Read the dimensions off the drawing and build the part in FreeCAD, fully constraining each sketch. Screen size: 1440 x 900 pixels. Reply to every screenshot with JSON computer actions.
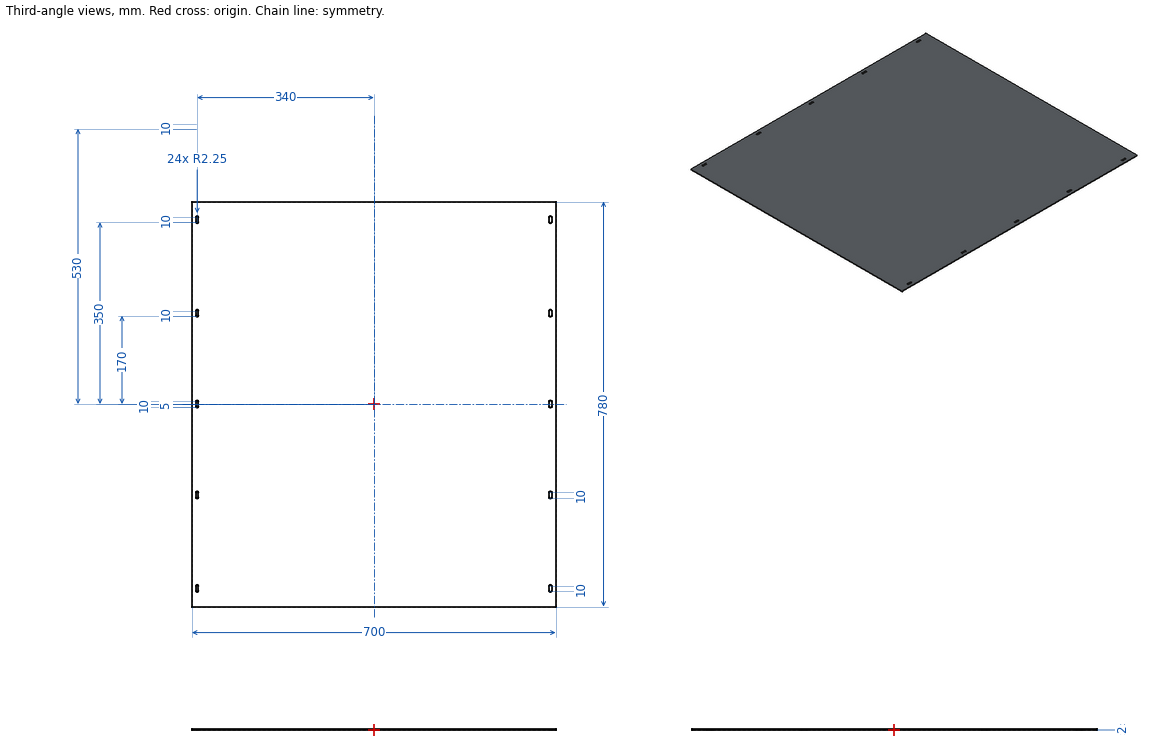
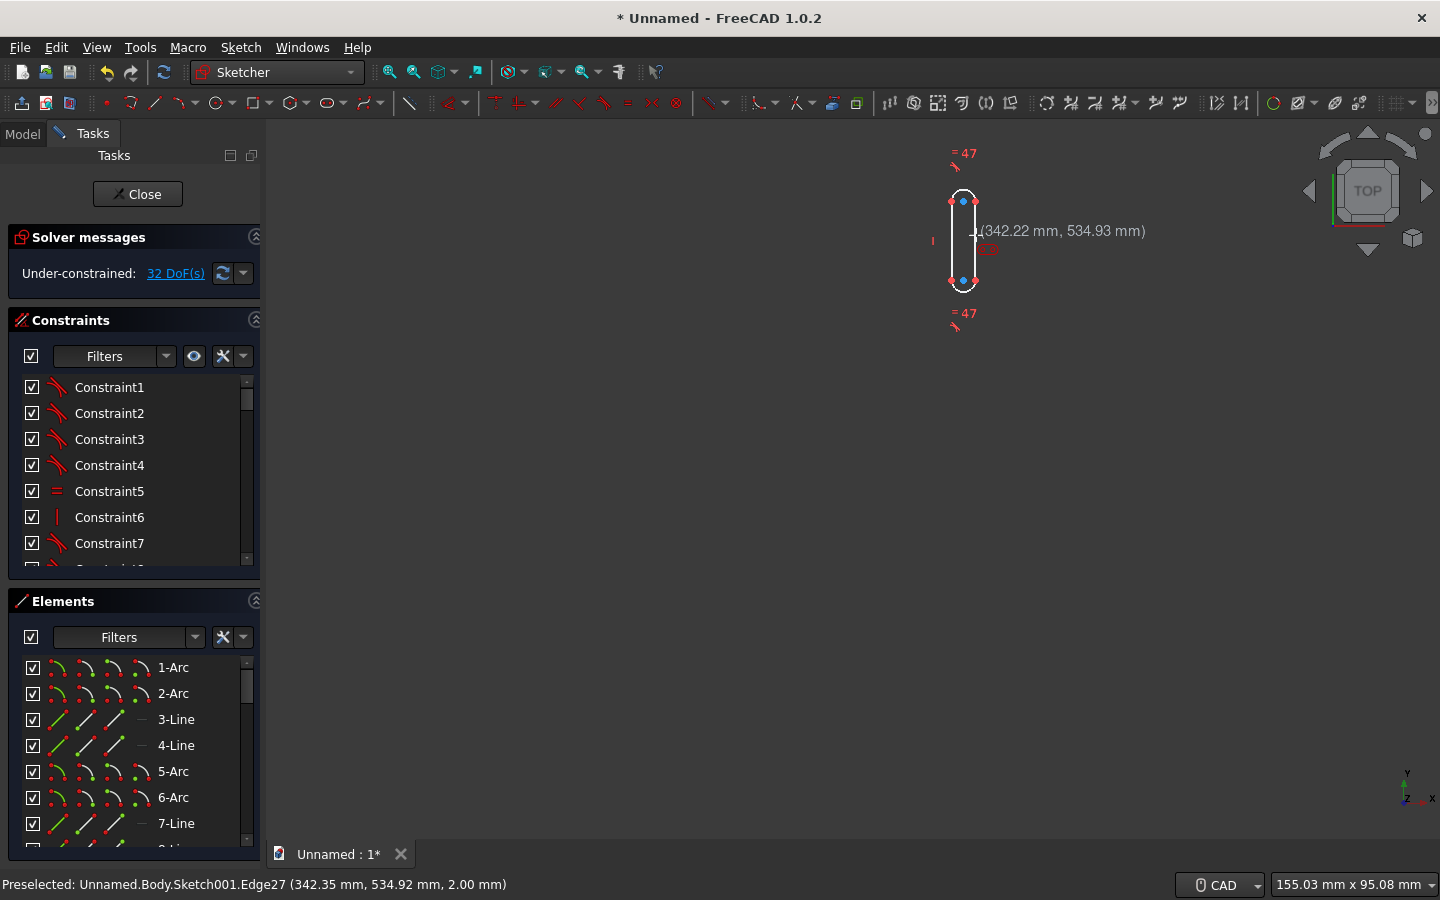
{"action": "scroll", "coordinate": [977, 228], "scroll_direction": "down", "scroll_amount": 13}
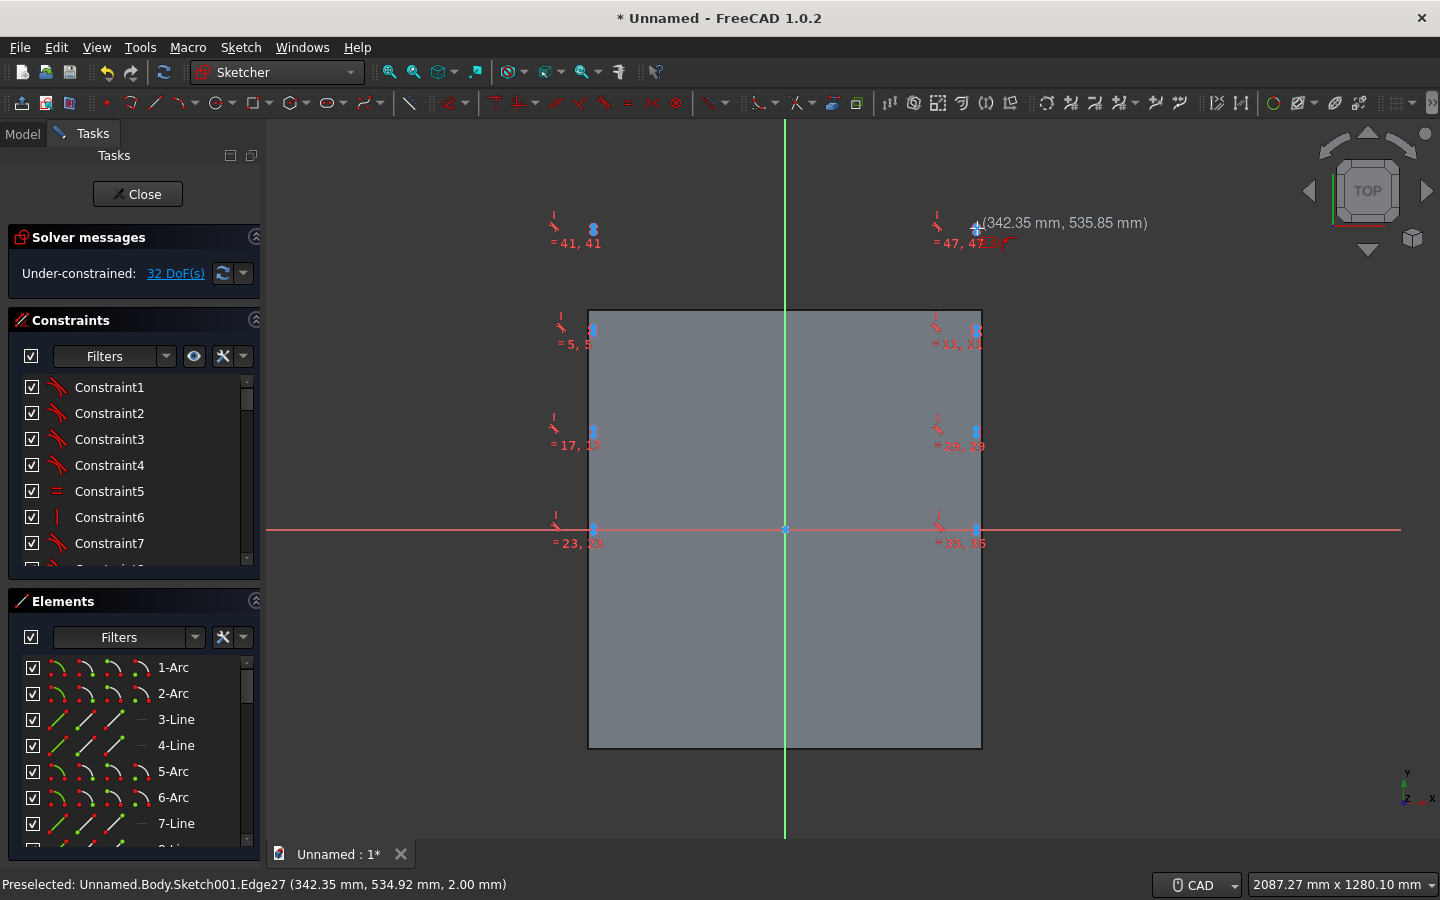
{"action": "scroll", "coordinate": [976, 631], "scroll_direction": "up", "scroll_amount": 15}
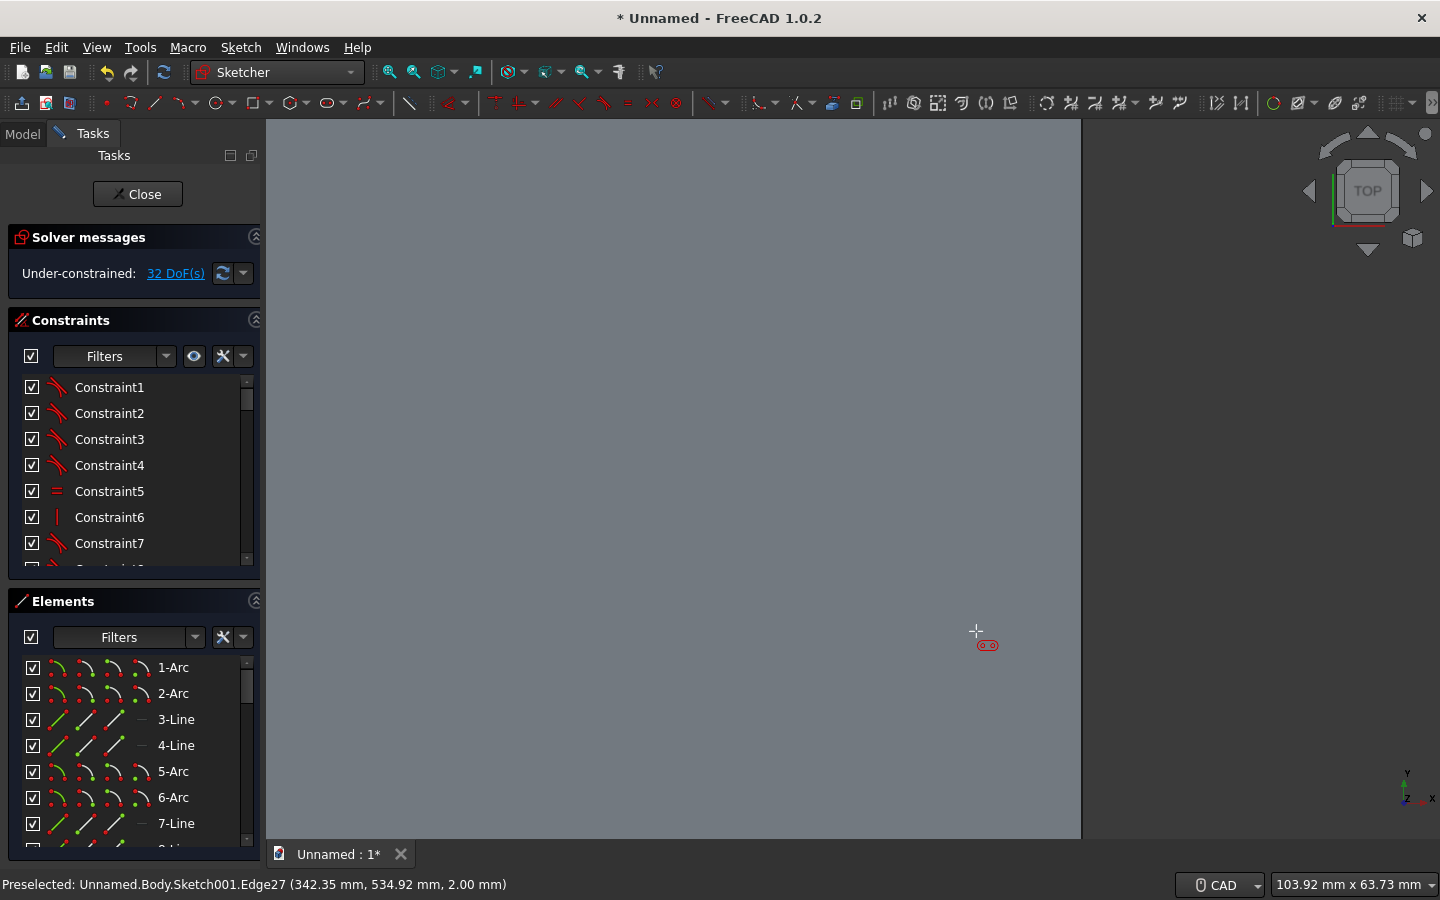
{"action": "scroll", "coordinate": [976, 632], "scroll_direction": "down", "scroll_amount": 15}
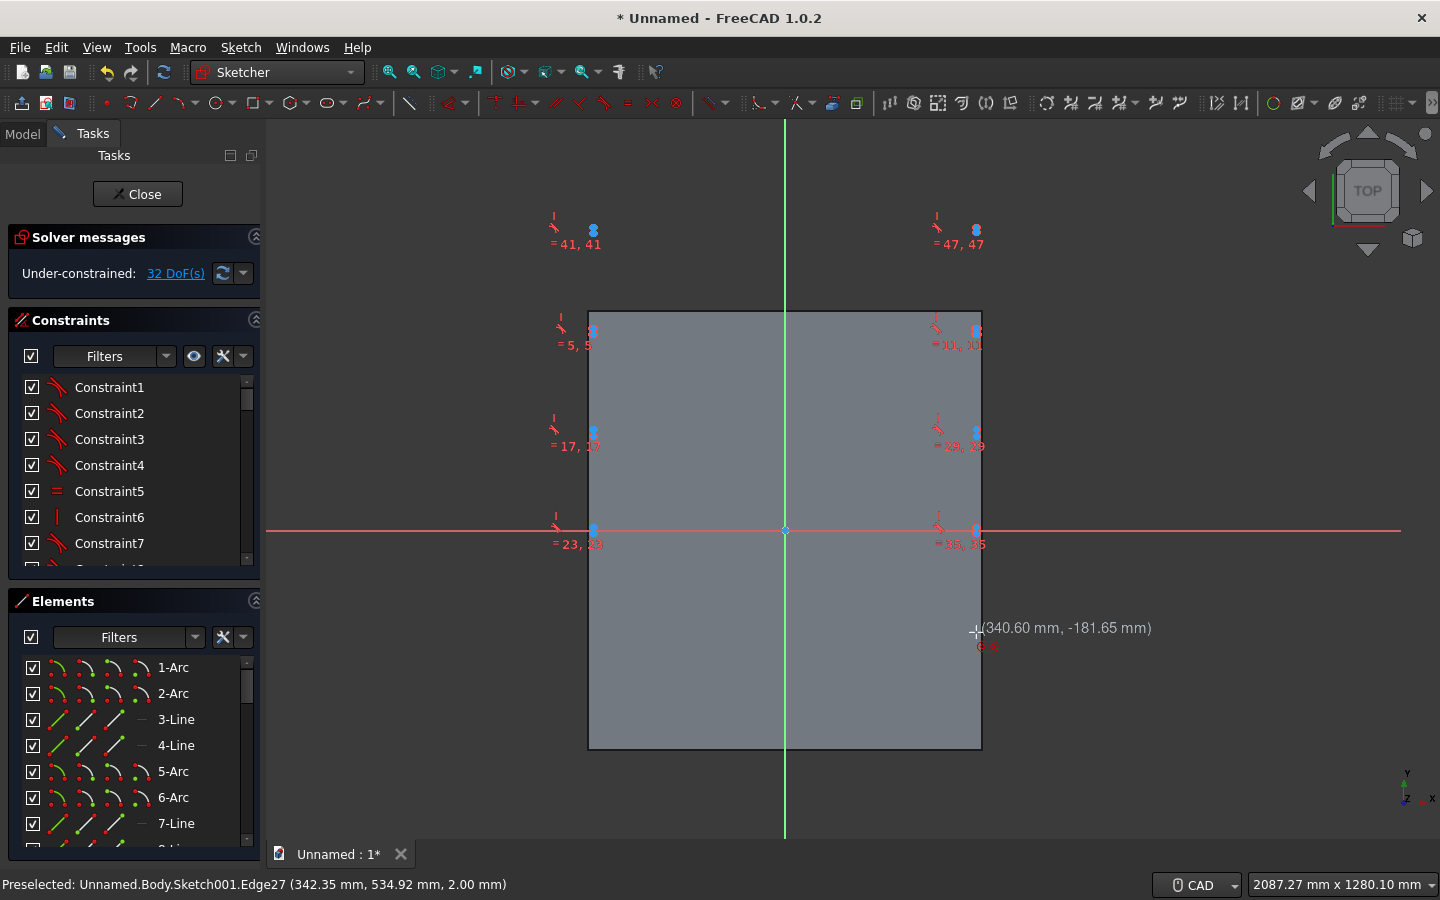
{"action": "left_click", "coordinate": [976, 632]}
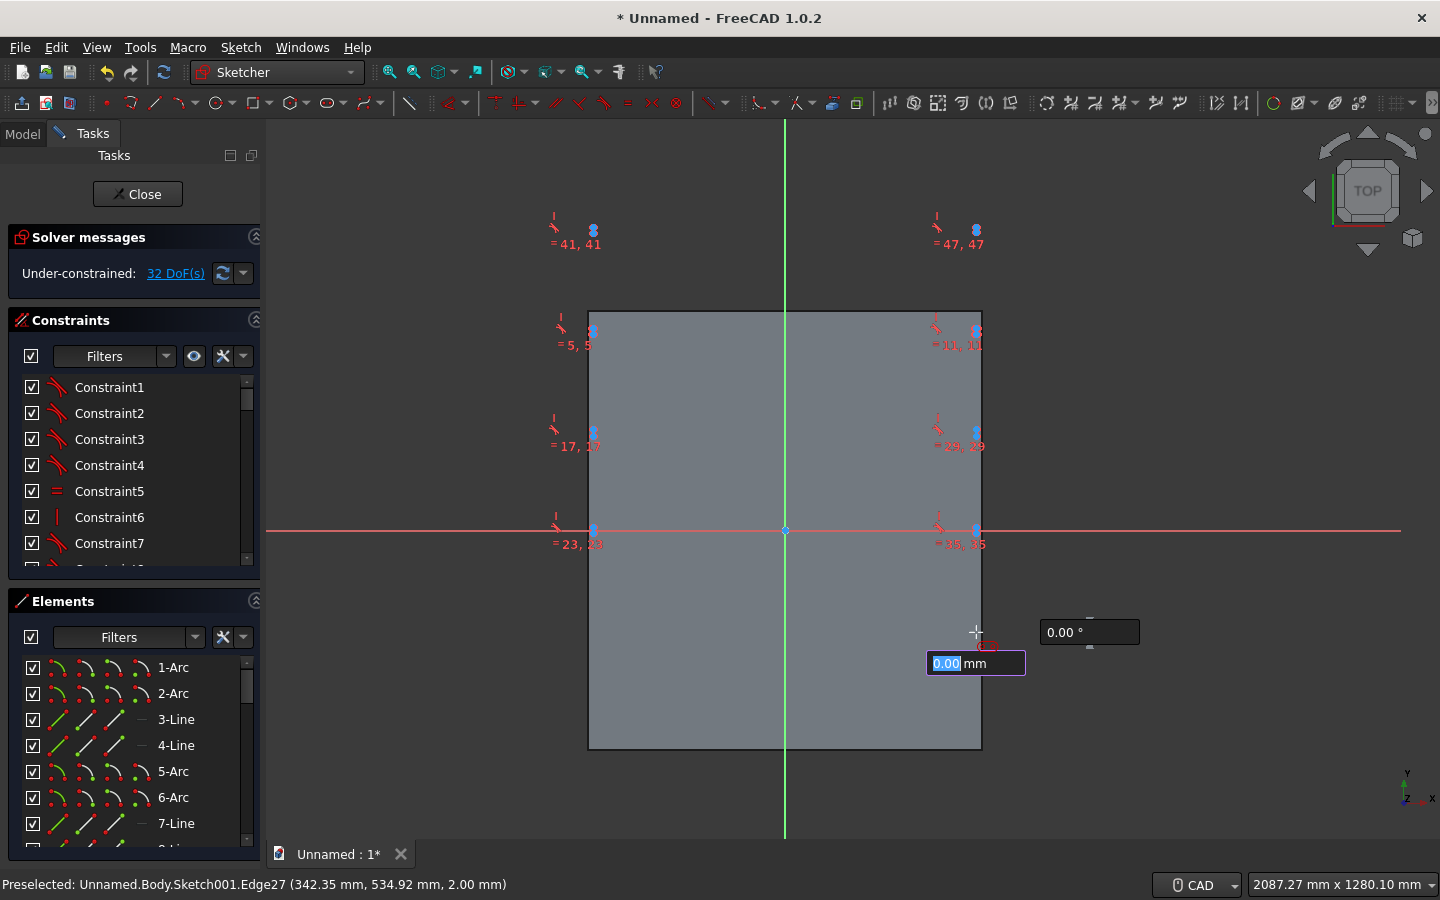
{"action": "scroll", "coordinate": [976, 626], "scroll_direction": "up", "scroll_amount": 6}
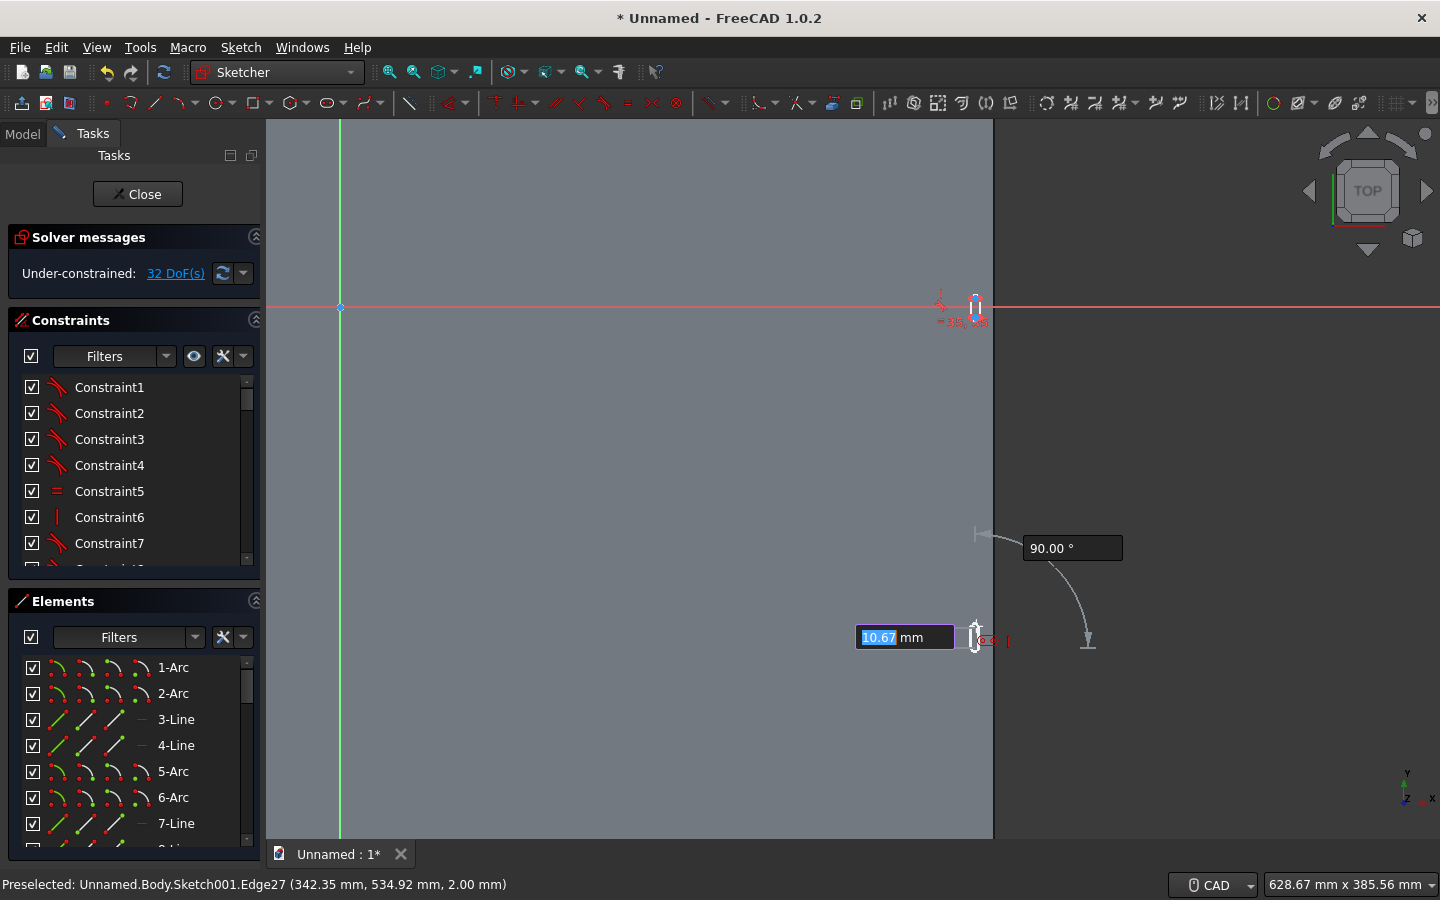
{"action": "left_click", "coordinate": [975, 625]}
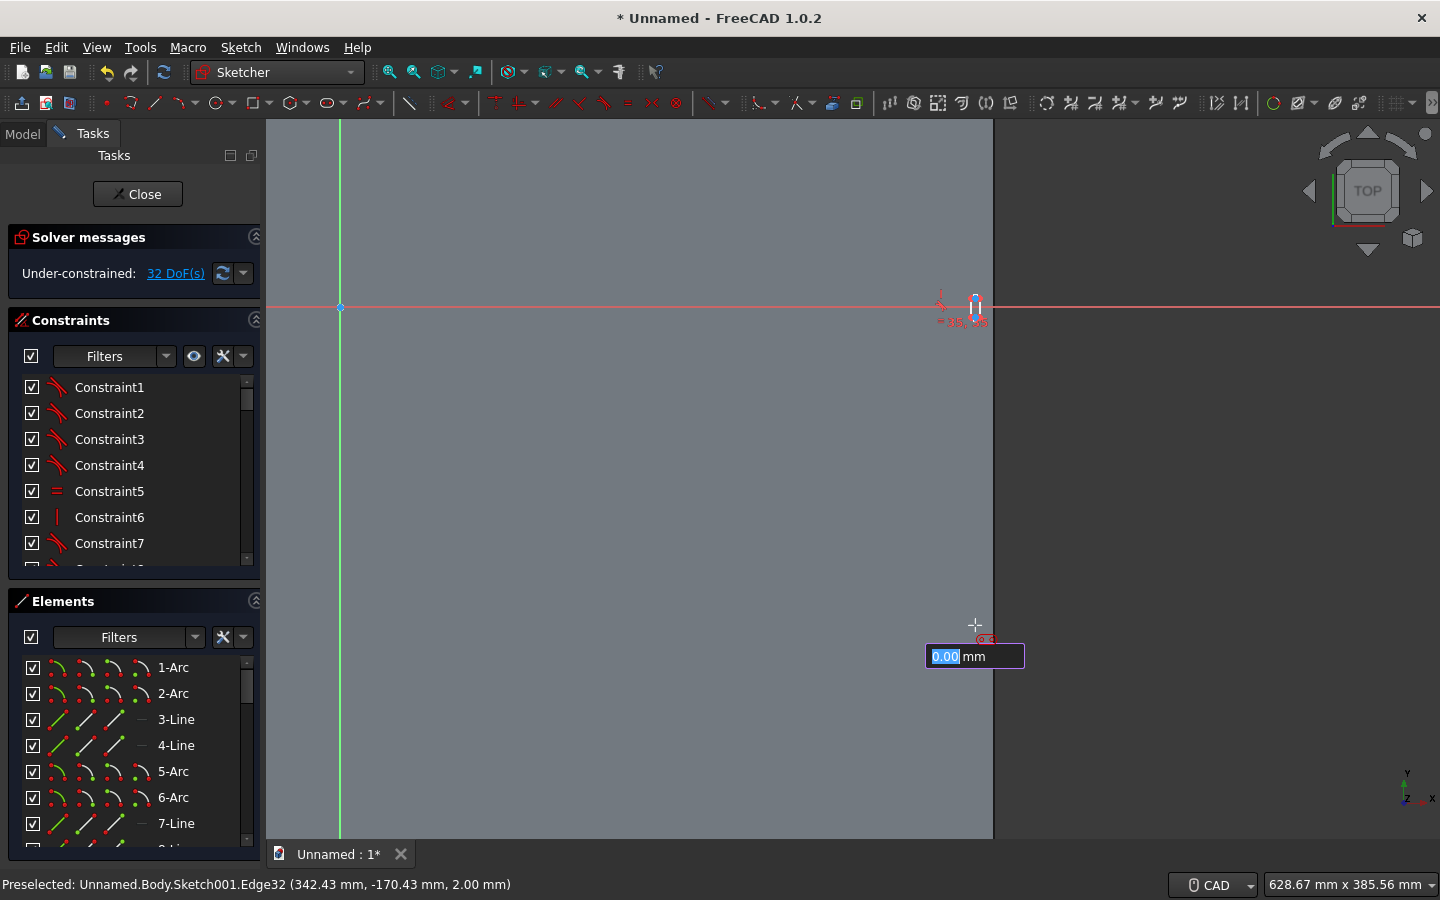
{"action": "scroll", "coordinate": [980, 634], "scroll_direction": "up", "scroll_amount": 7}